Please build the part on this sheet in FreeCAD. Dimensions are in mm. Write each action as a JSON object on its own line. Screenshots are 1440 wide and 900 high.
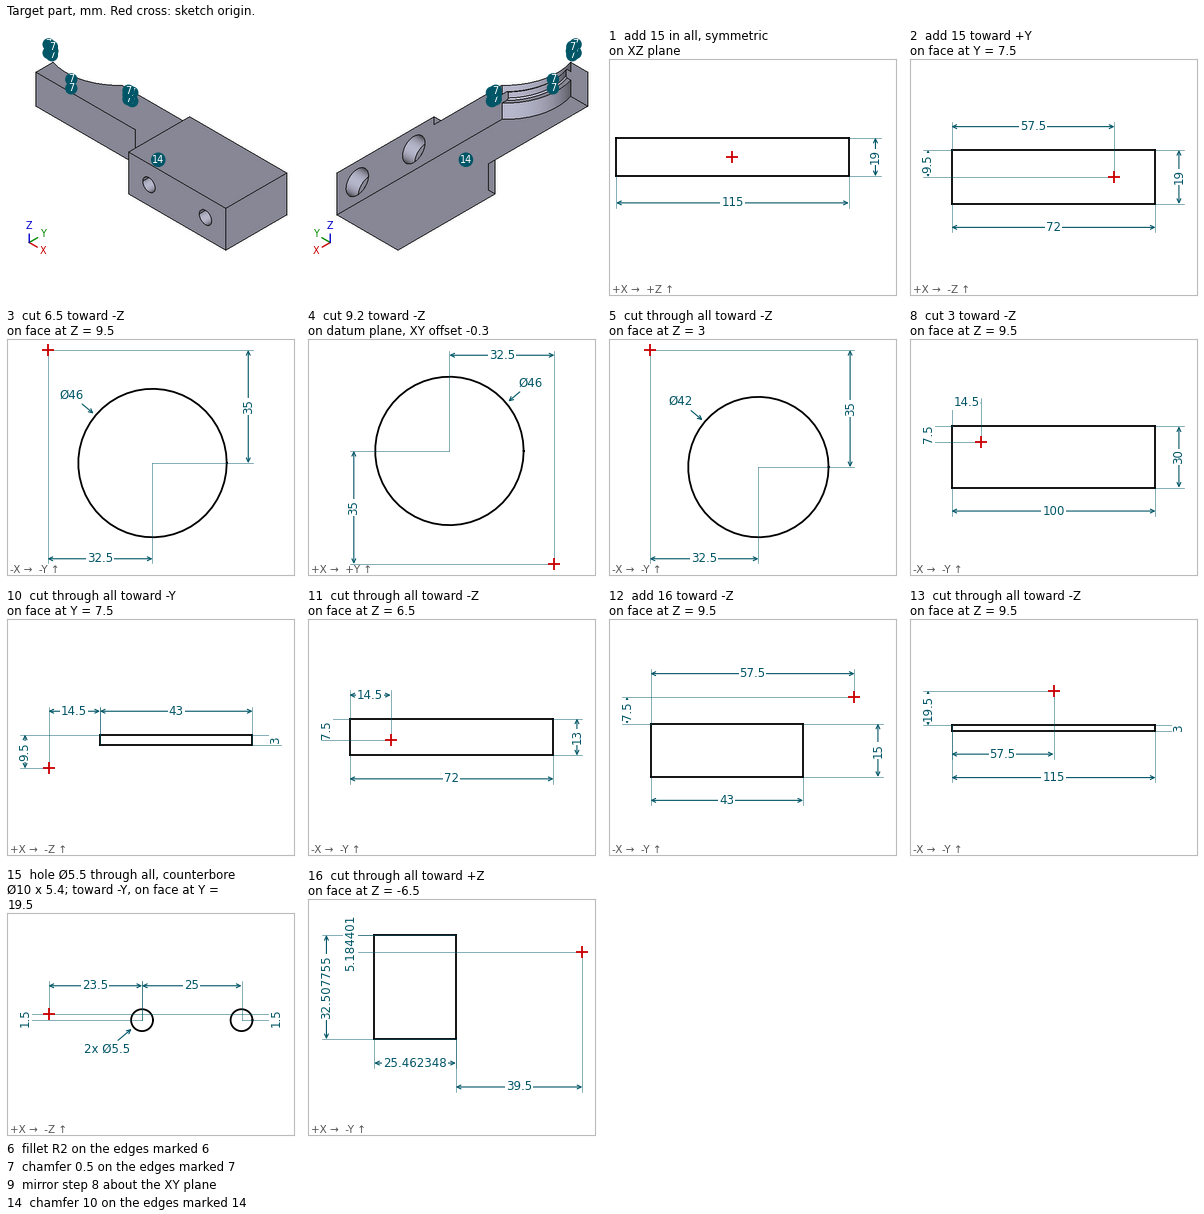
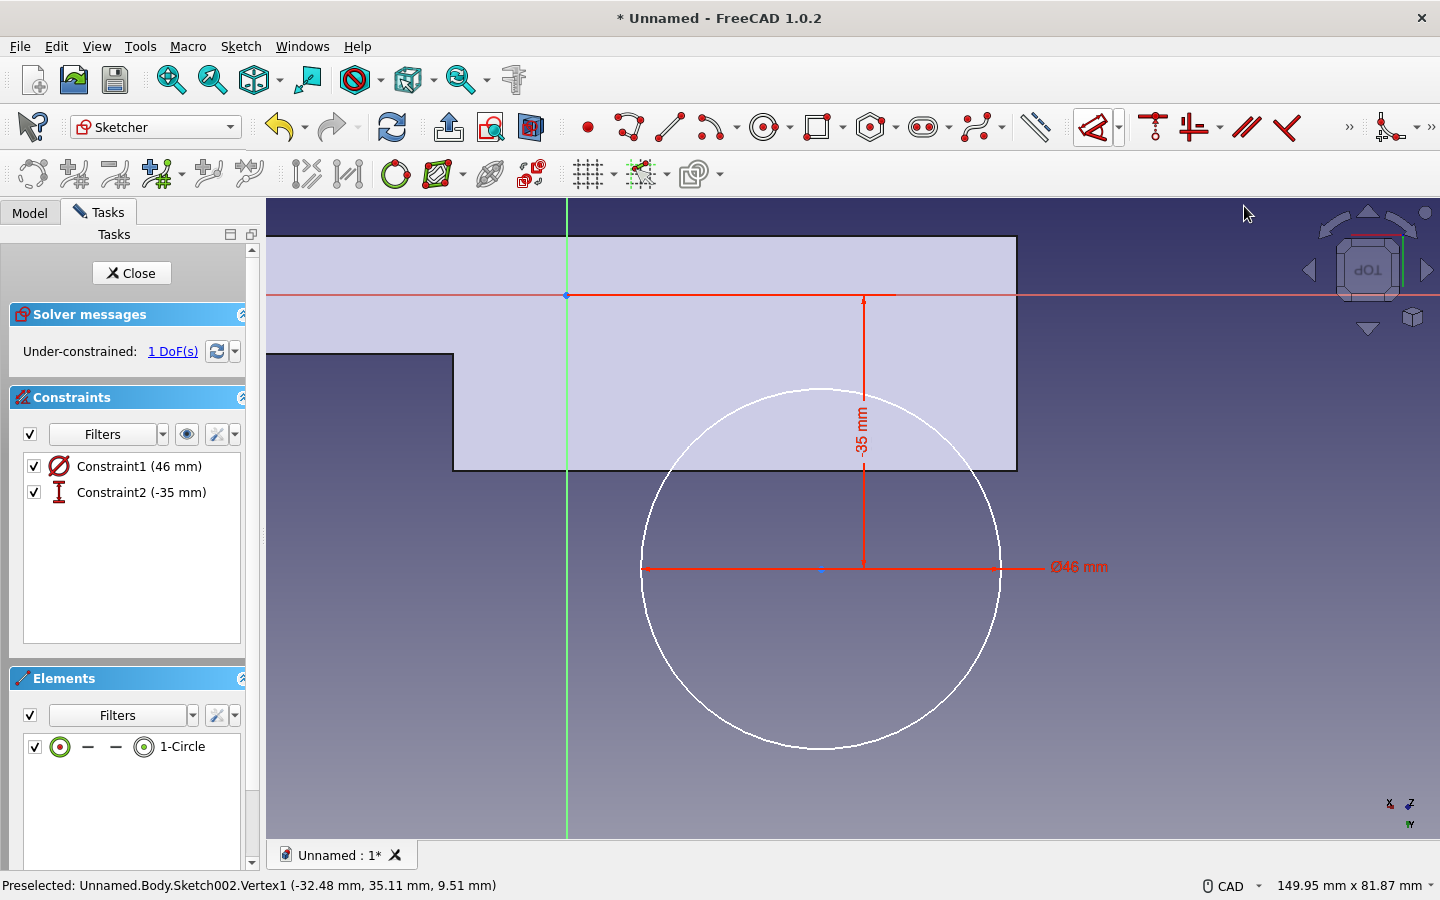
{"action": "left_click", "coordinate": [821, 569]}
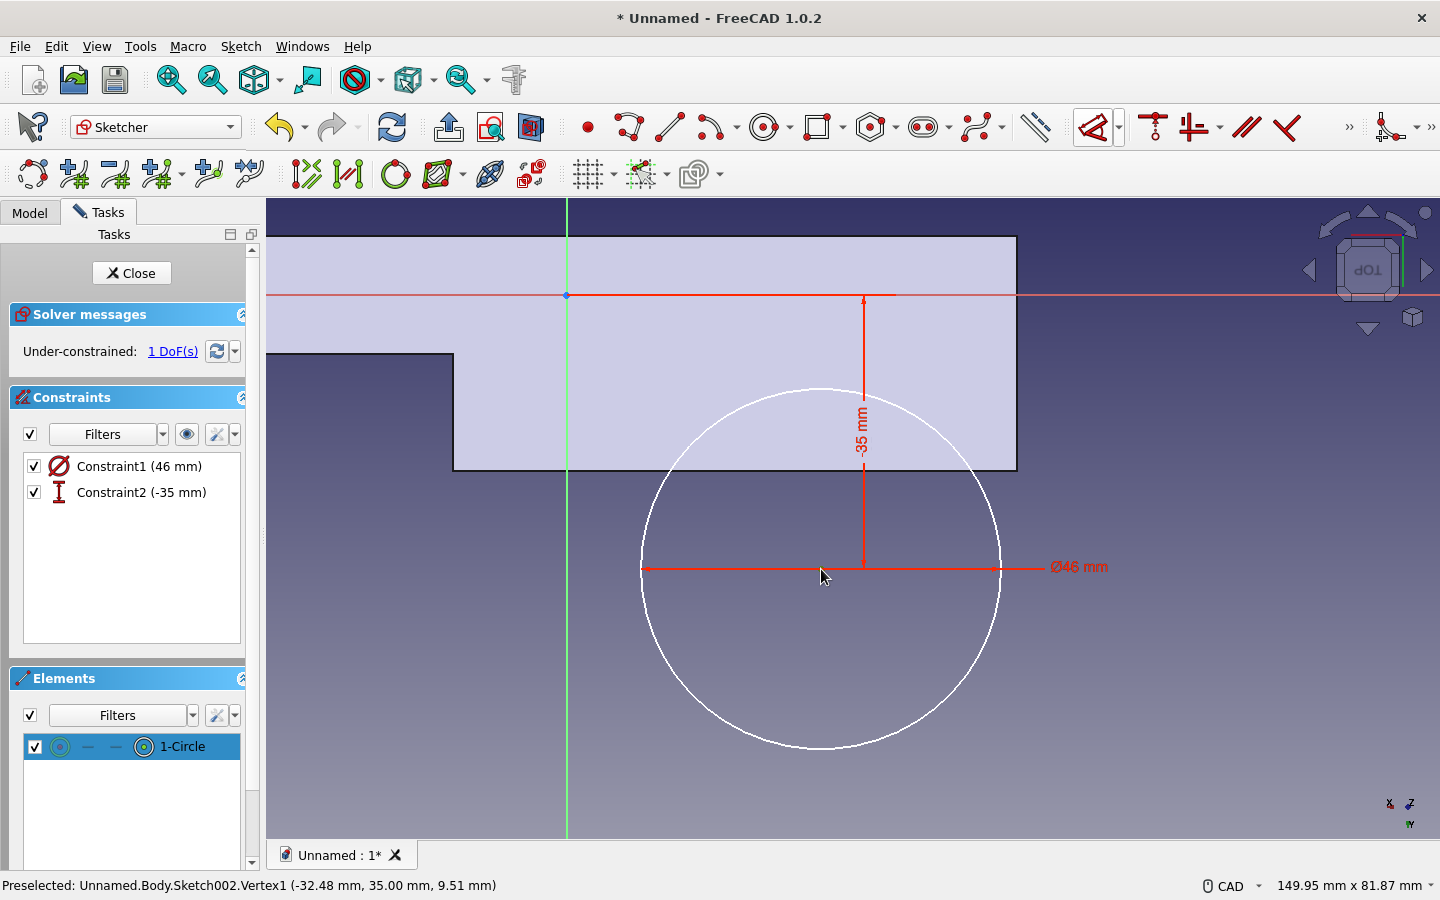
{"action": "key", "text": "l"}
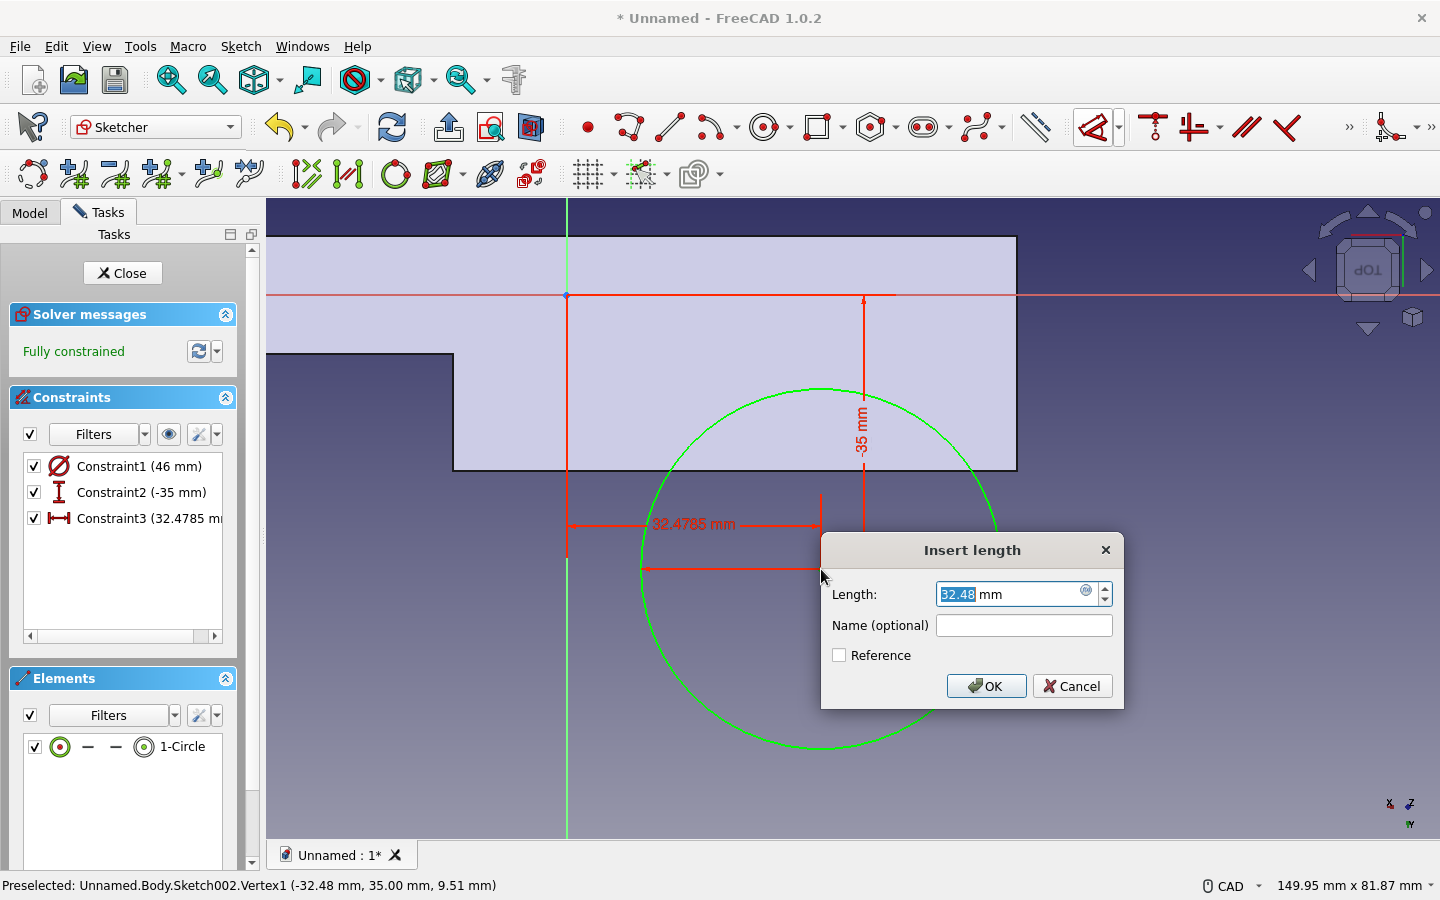
{"action": "type", "text": "32.5"}
{"action": "key", "text": "Return"}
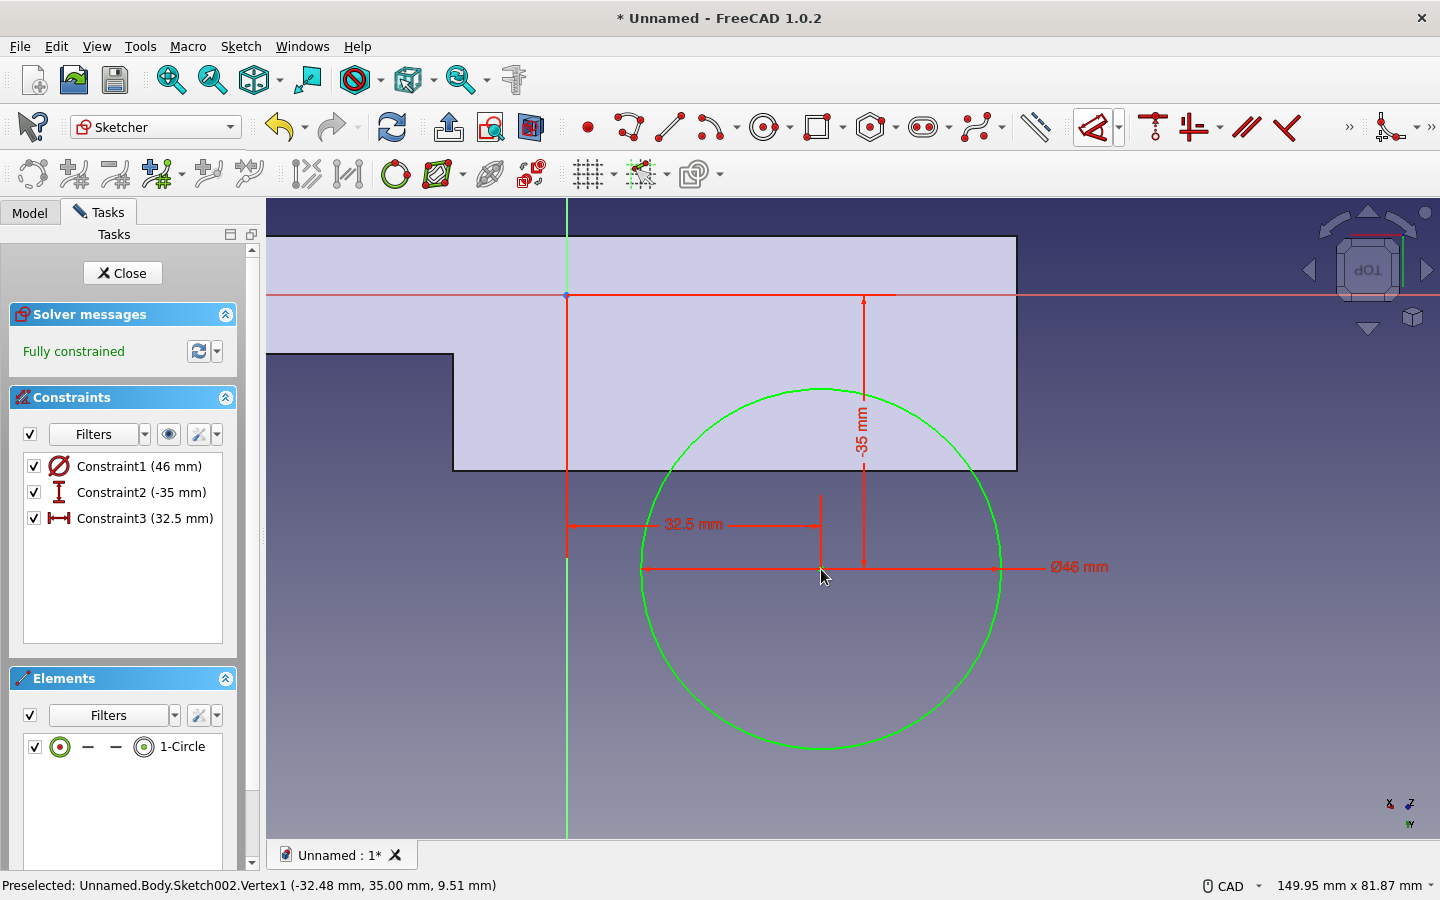
{"action": "left_click", "coordinate": [123, 273]}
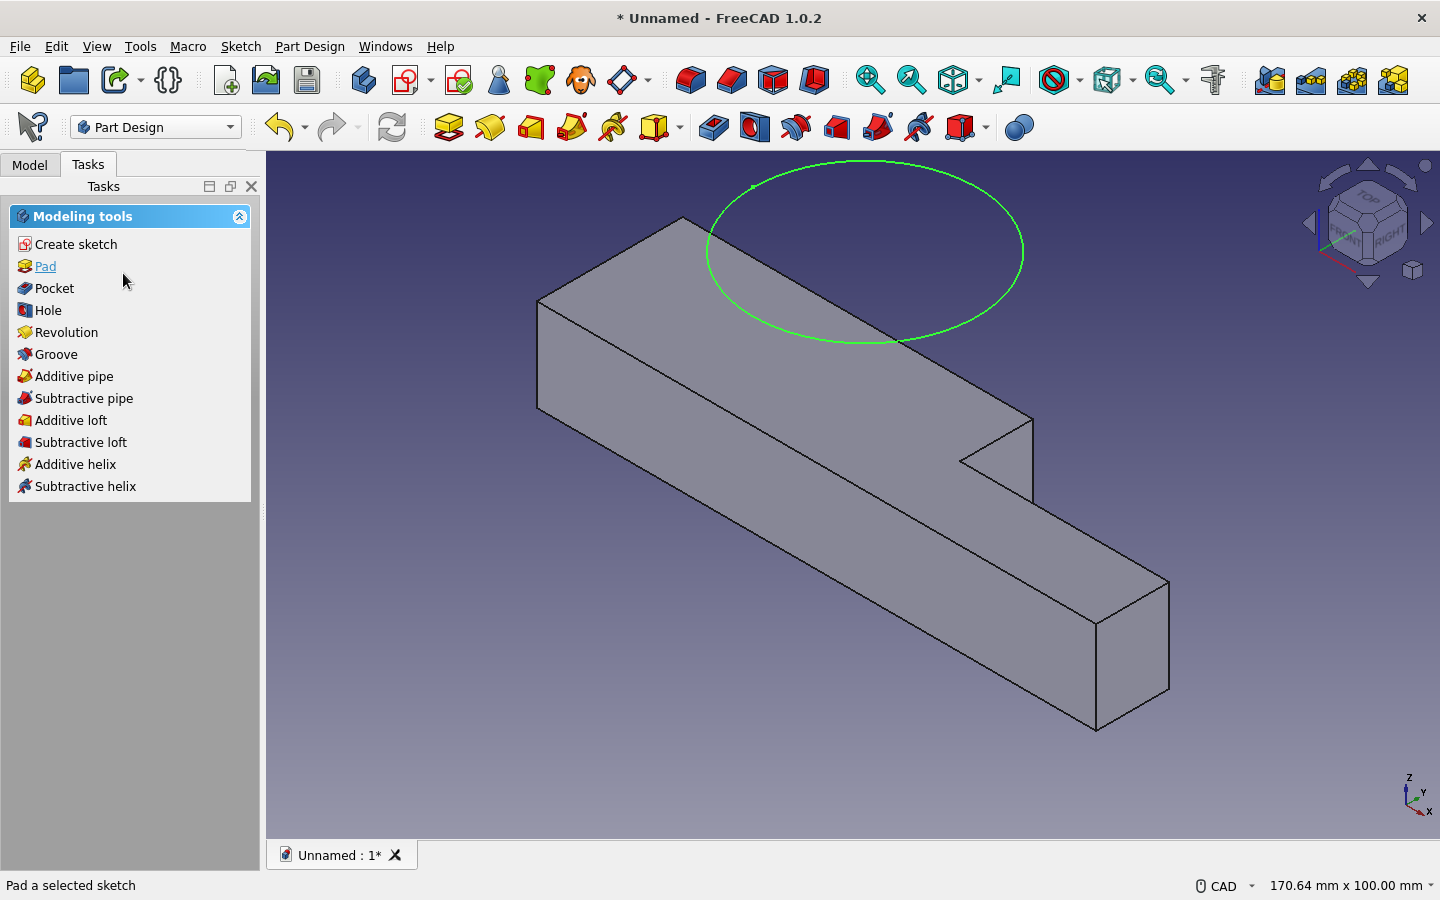
{"action": "left_click", "coordinate": [714, 128]}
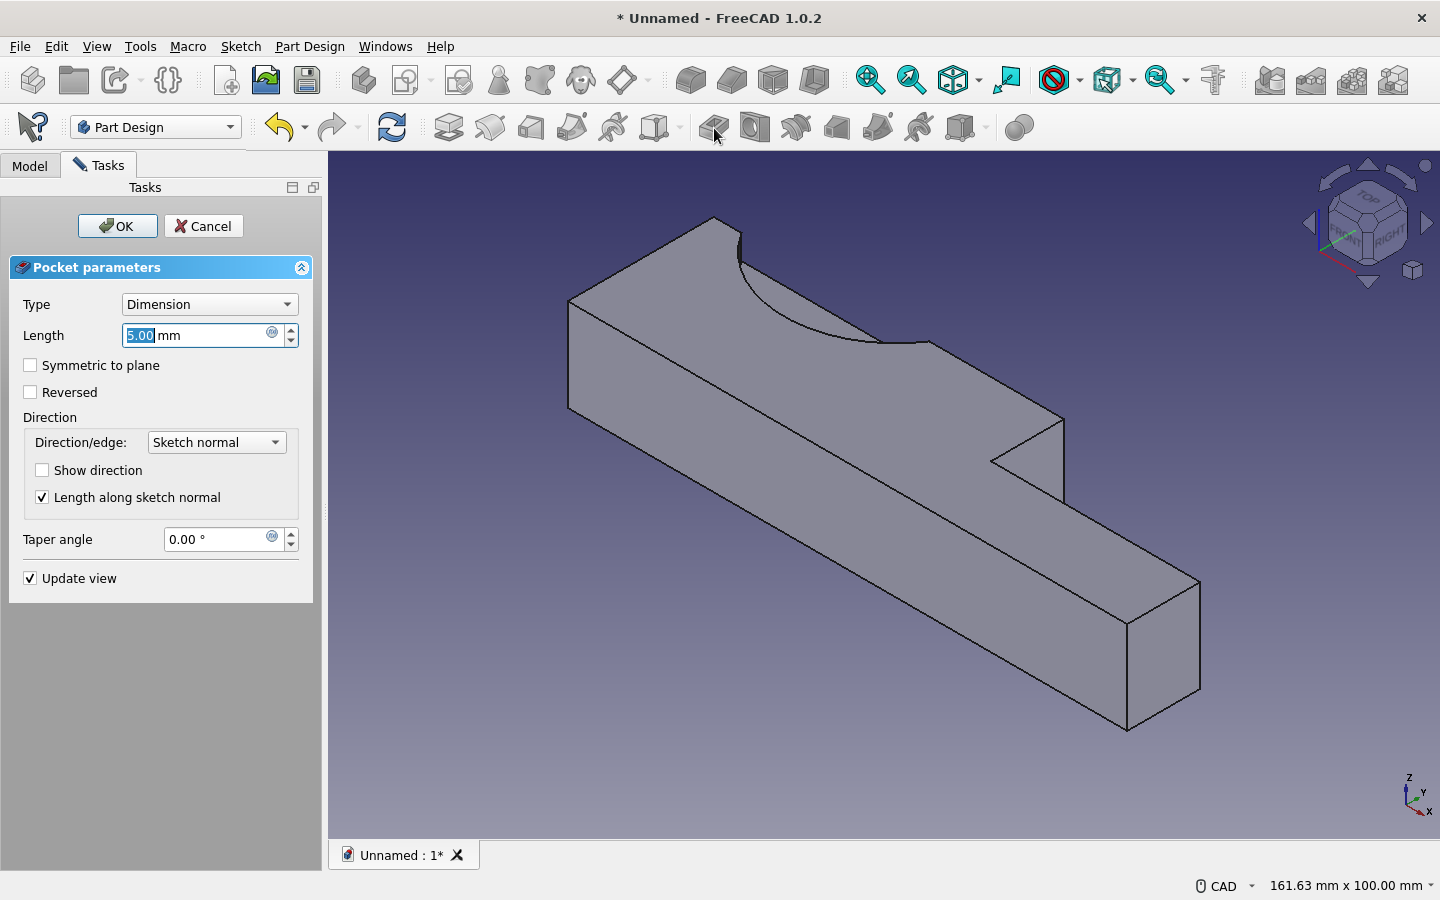
{"action": "type", "text": "6.5"}
{"action": "key", "text": "Tab"}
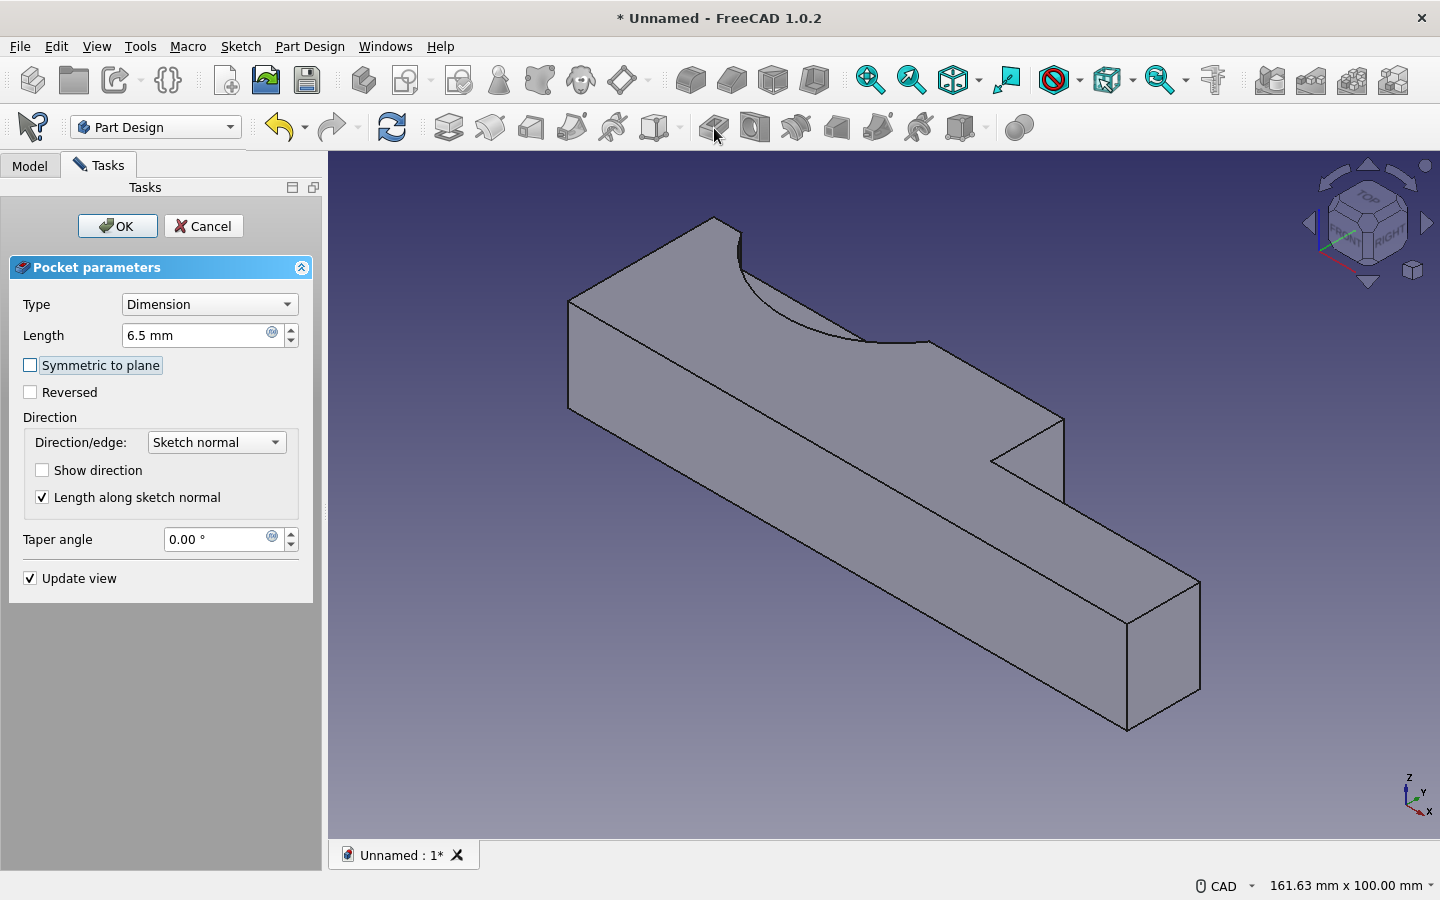
{"action": "left_click", "coordinate": [118, 226]}